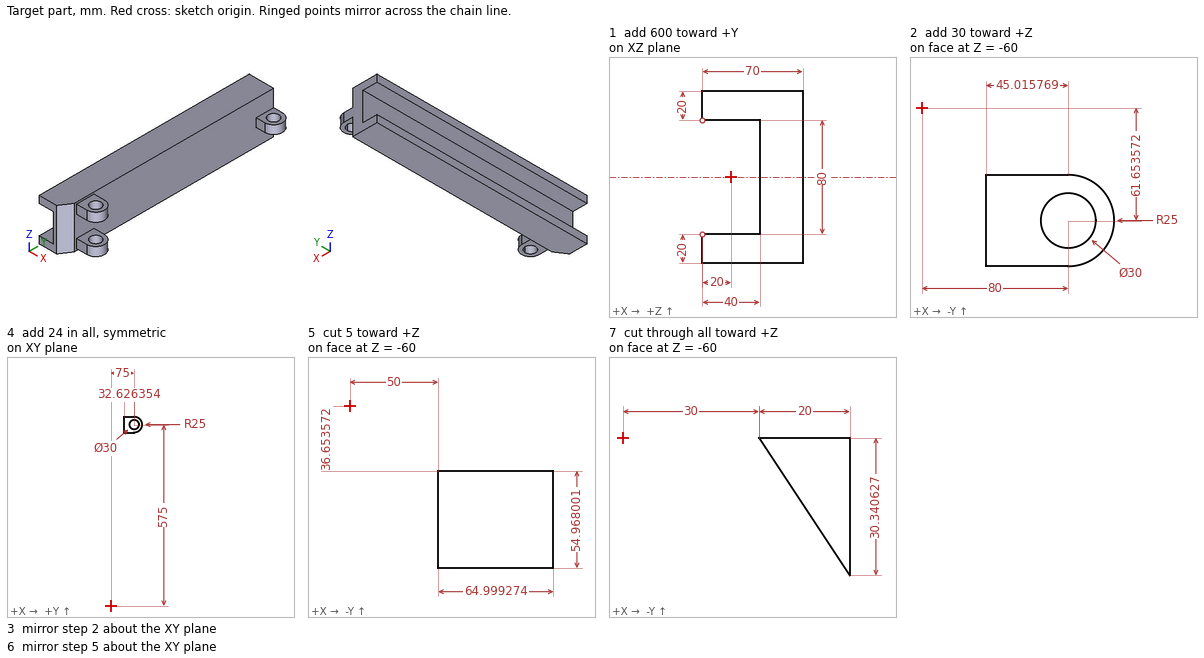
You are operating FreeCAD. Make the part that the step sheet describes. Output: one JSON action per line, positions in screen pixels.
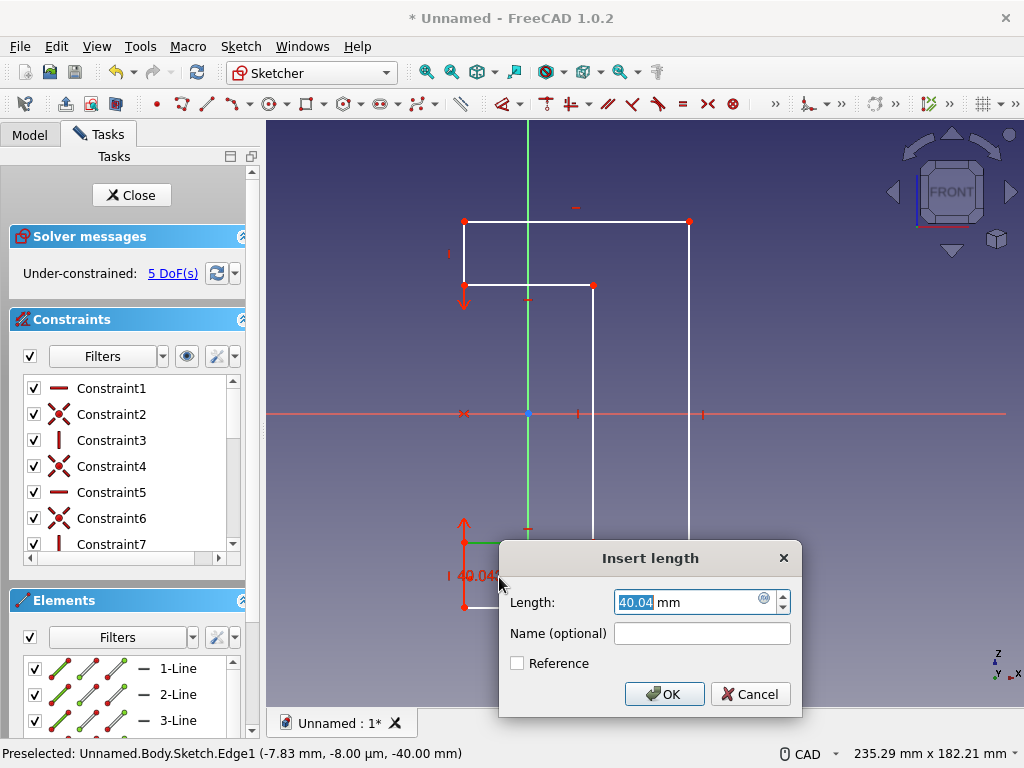
{"action": "type", "text": "40"}
{"action": "key", "text": "Return"}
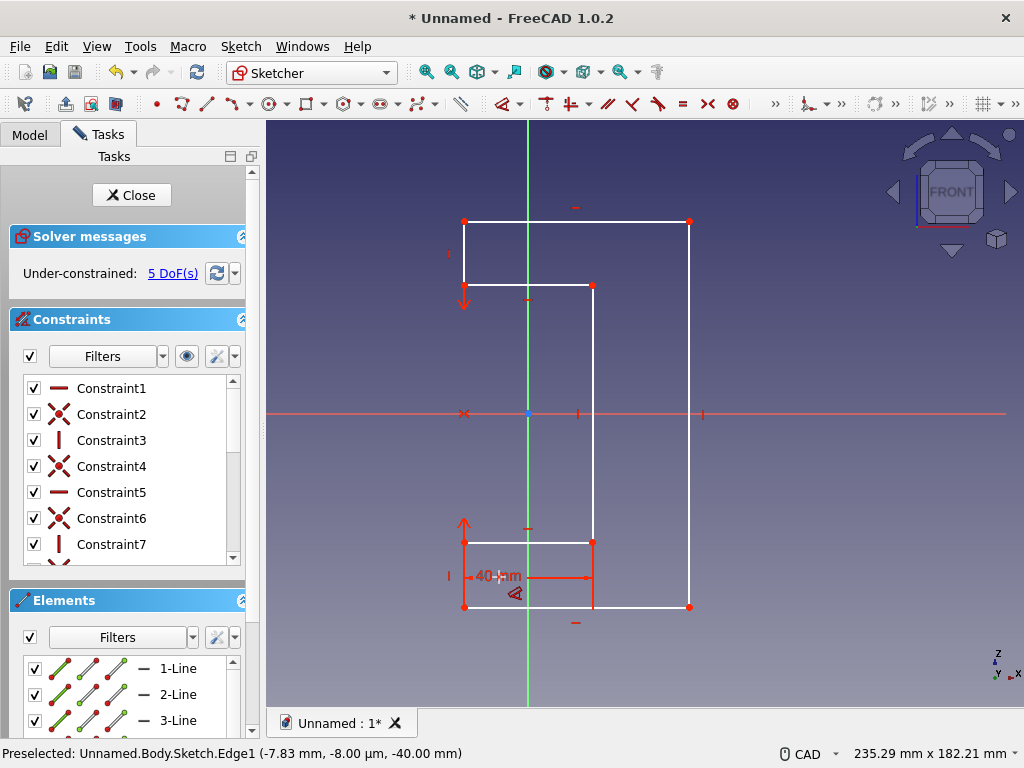
{"action": "left_click", "coordinate": [593, 465]}
{"action": "left_click", "coordinate": [627, 355]}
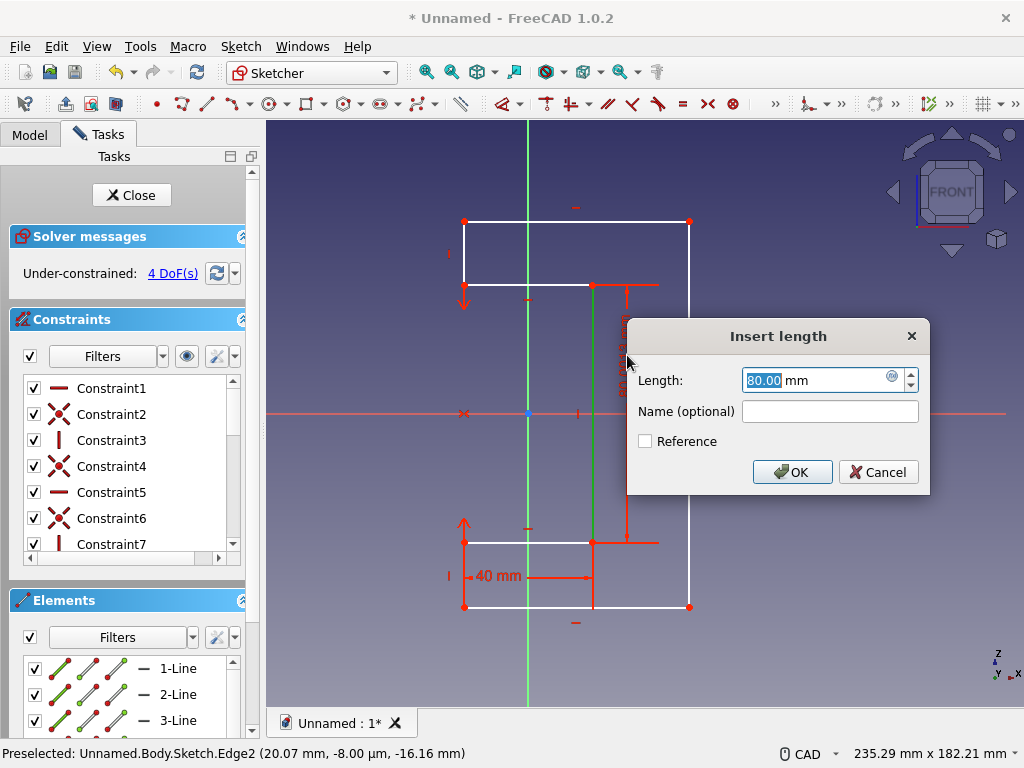
{"action": "type", "text": "80"}
{"action": "key", "text": "Return"}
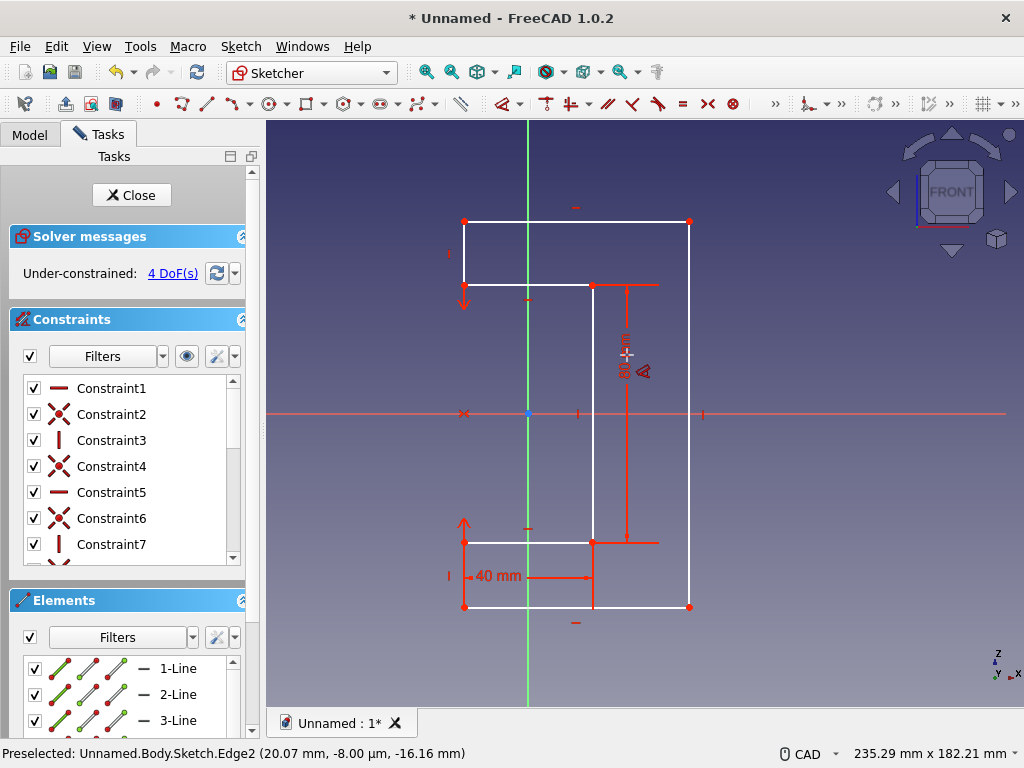
{"action": "left_click", "coordinate": [464, 266]}
{"action": "left_click", "coordinate": [430, 254]}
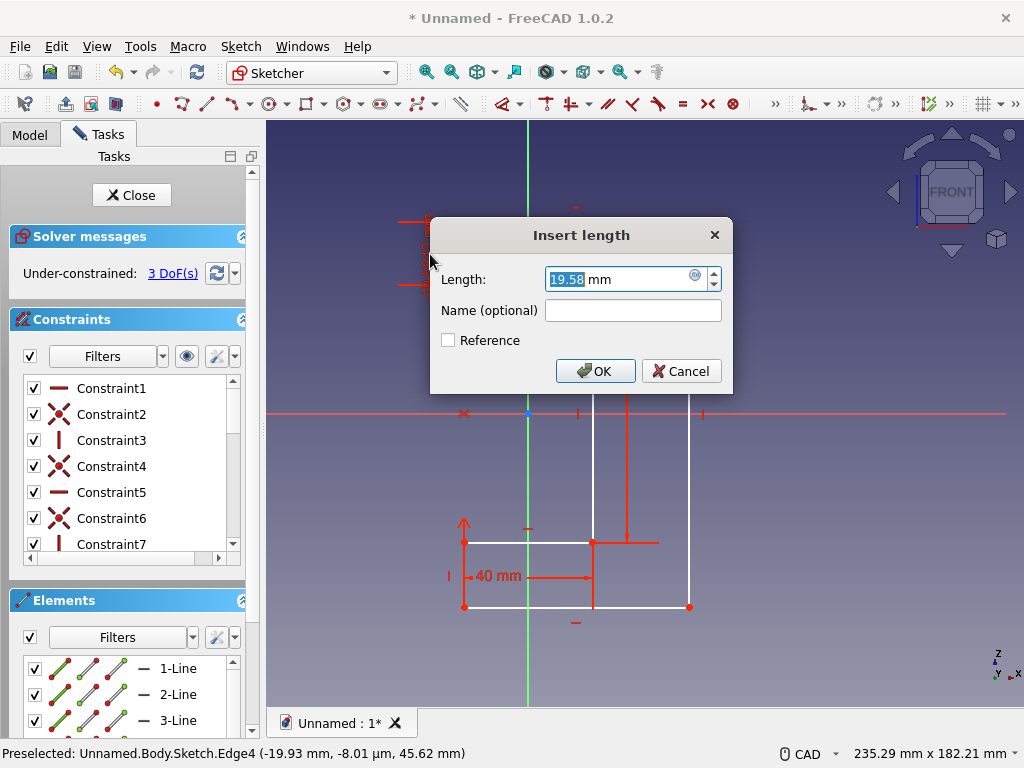
{"action": "type", "text": "20"}
{"action": "key", "text": "Return"}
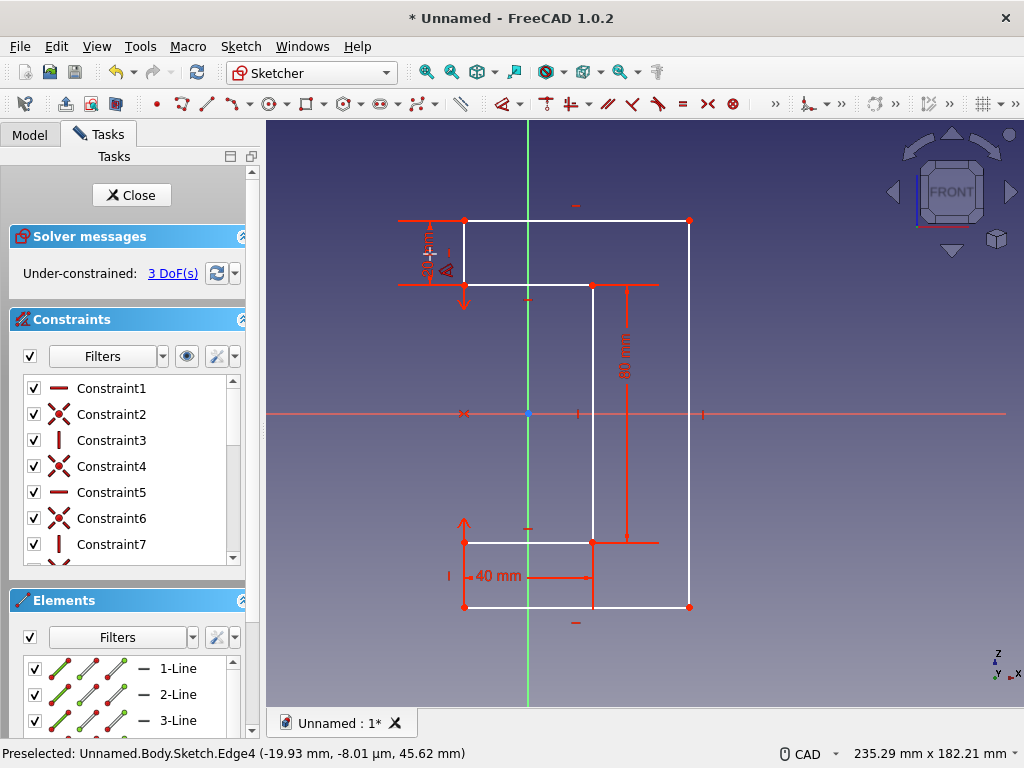
{"action": "left_click", "coordinate": [531, 221]}
{"action": "left_click", "coordinate": [576, 187]}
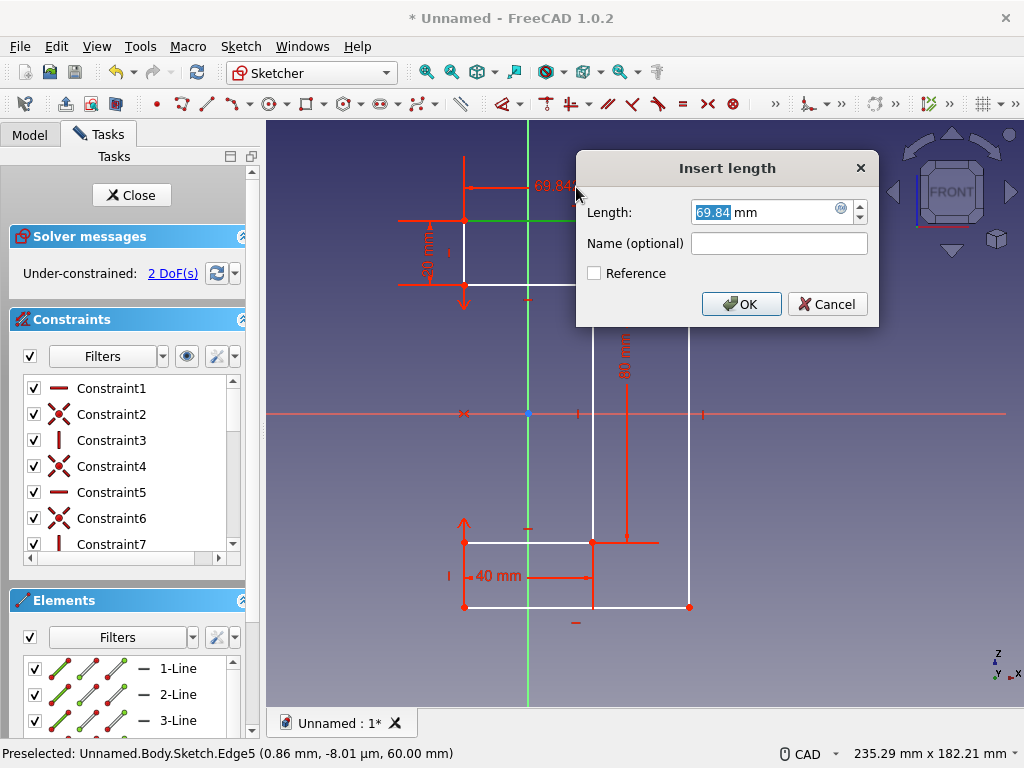
{"action": "type", "text": "70"}
{"action": "key", "text": "Return"}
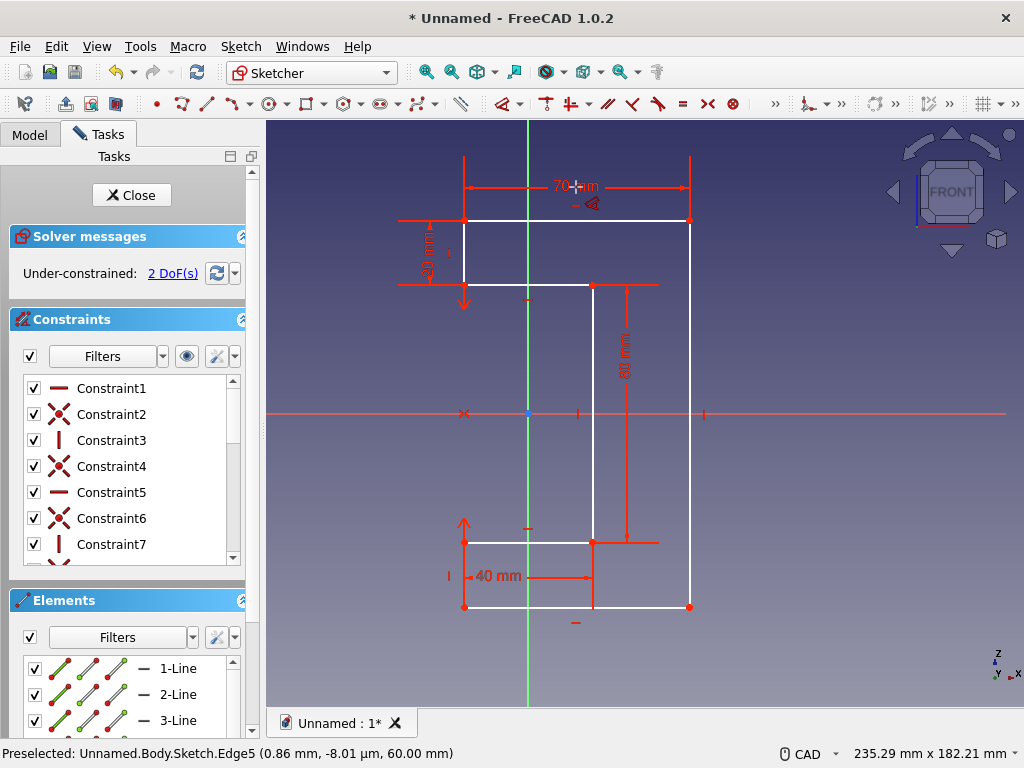
{"action": "left_click", "coordinate": [464, 588]}
{"action": "left_click", "coordinate": [430, 553]}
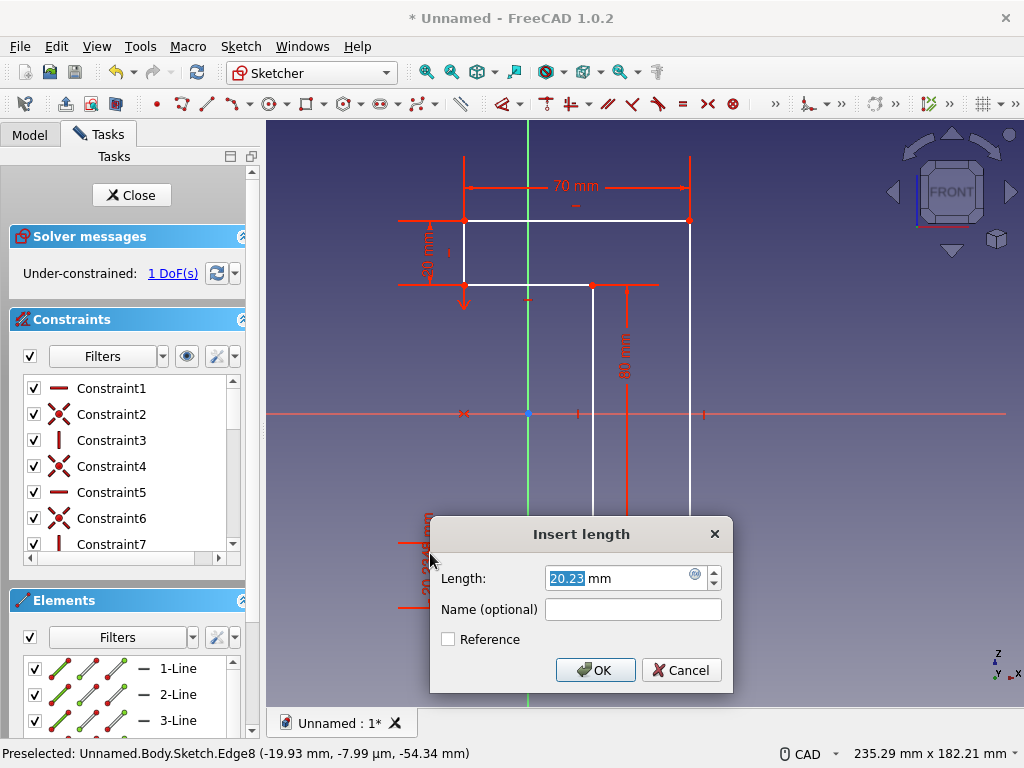
{"action": "type", "text": "20"}
{"action": "key", "text": "Return"}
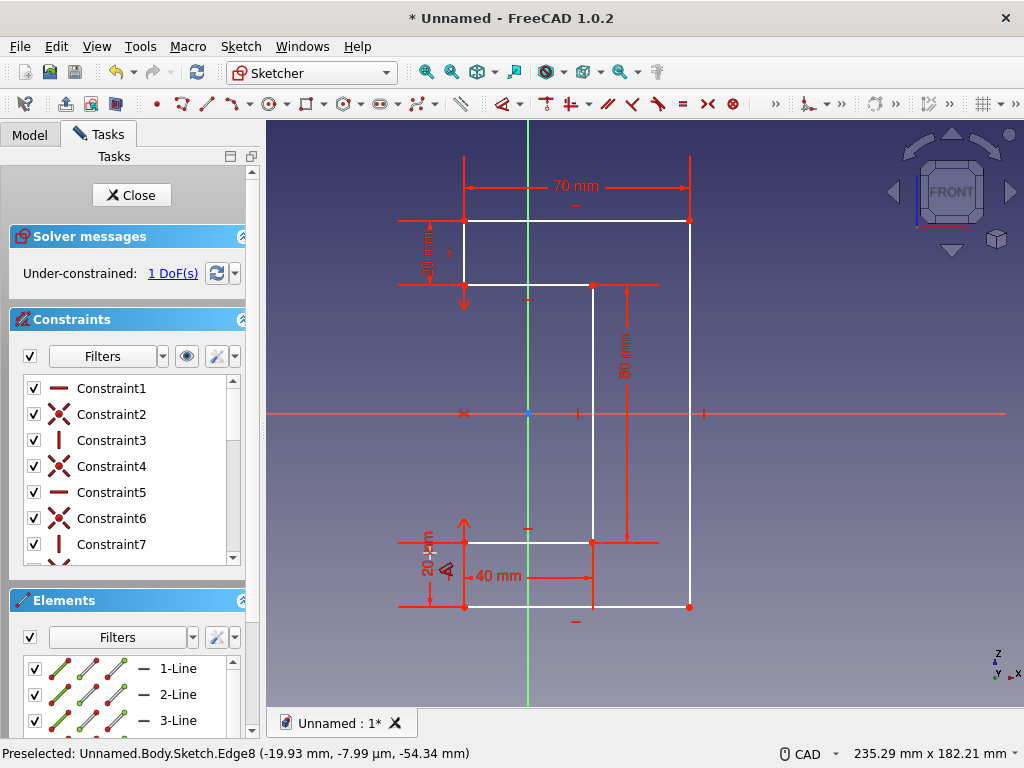
{"action": "left_click", "coordinate": [464, 543]}
{"action": "left_click", "coordinate": [496, 380]}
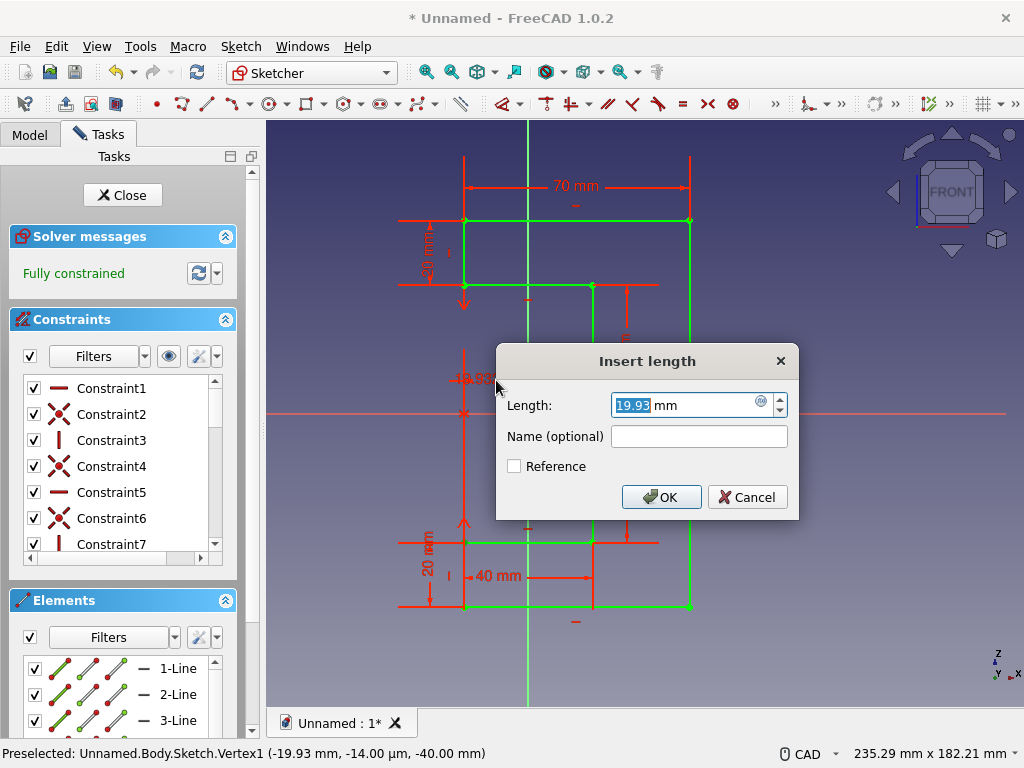
{"action": "type", "text": "20"}
{"action": "key", "text": "Return"}
{"action": "key", "text": "Escape"}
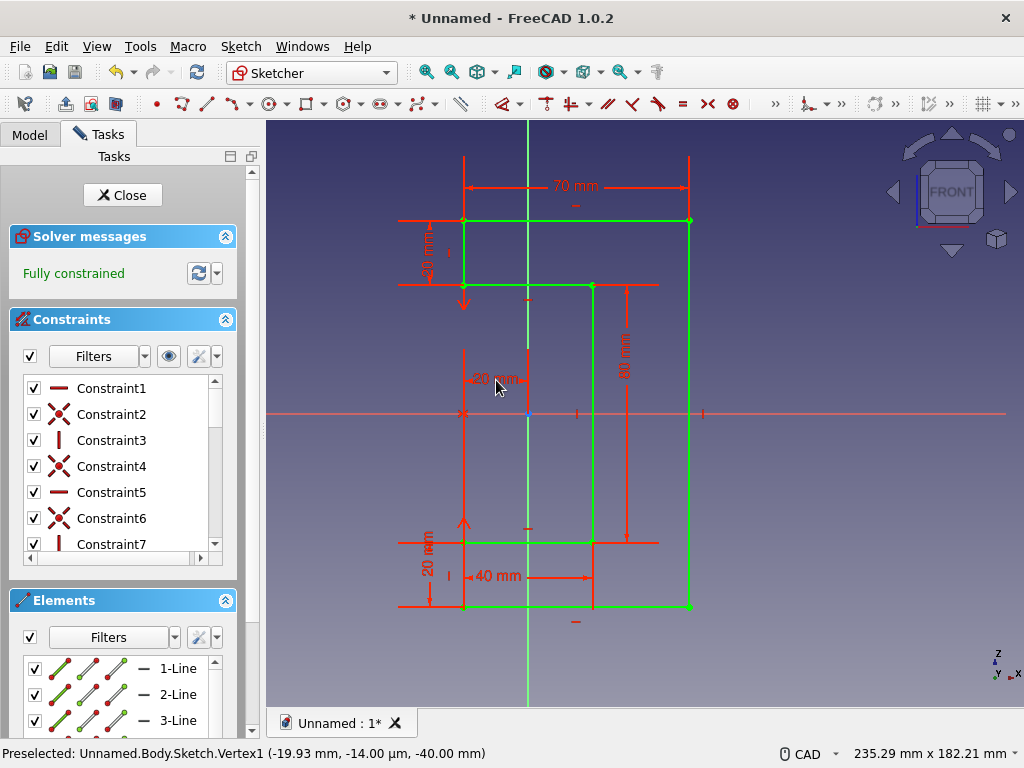
{"action": "left_click", "coordinate": [123, 195]}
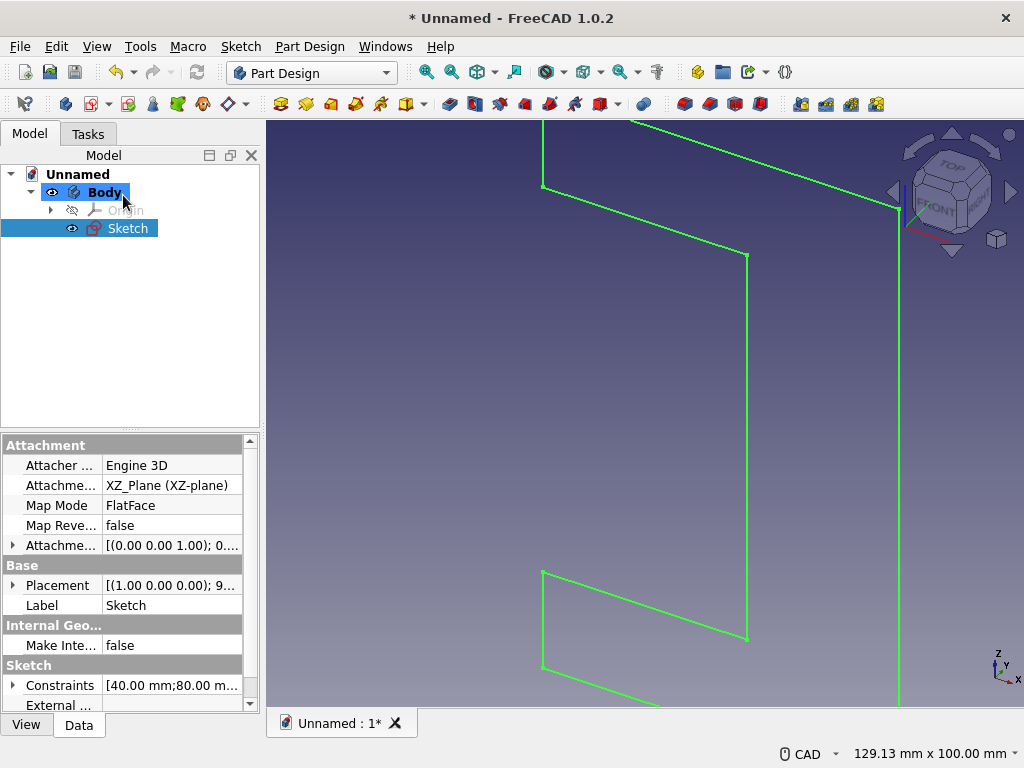
{"action": "left_click", "coordinate": [281, 104]}